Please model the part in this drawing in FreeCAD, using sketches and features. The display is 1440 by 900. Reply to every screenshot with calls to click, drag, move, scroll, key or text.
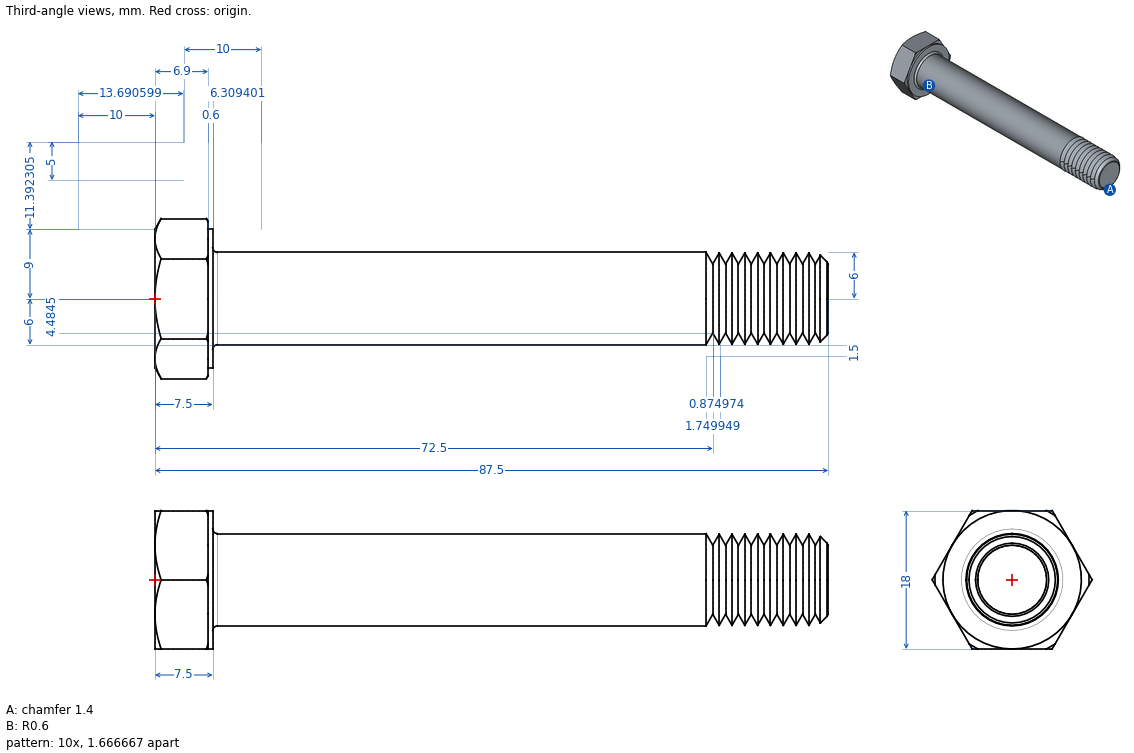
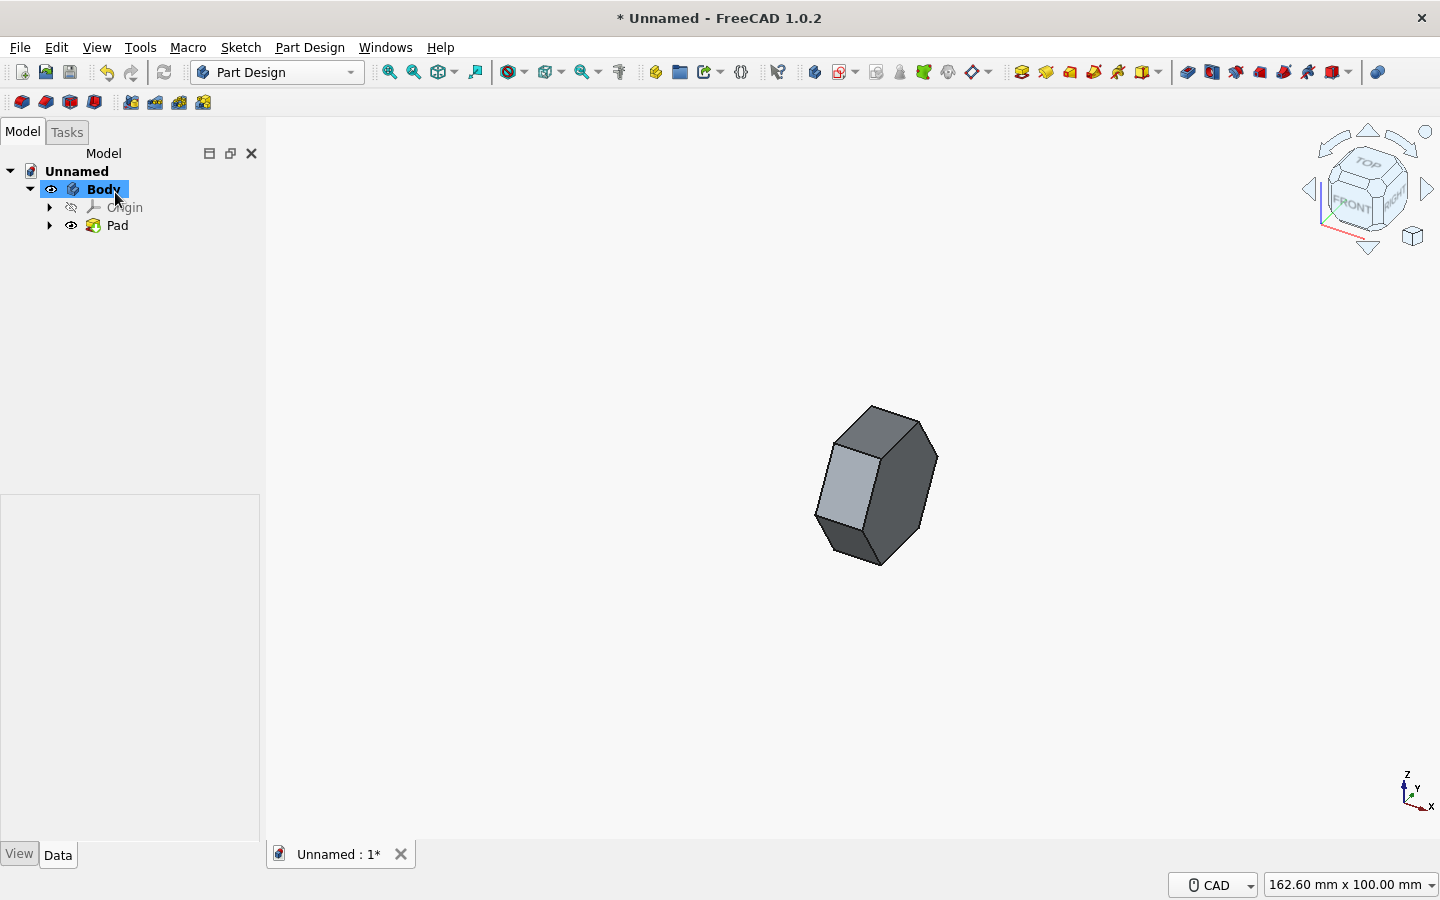
click(390, 72)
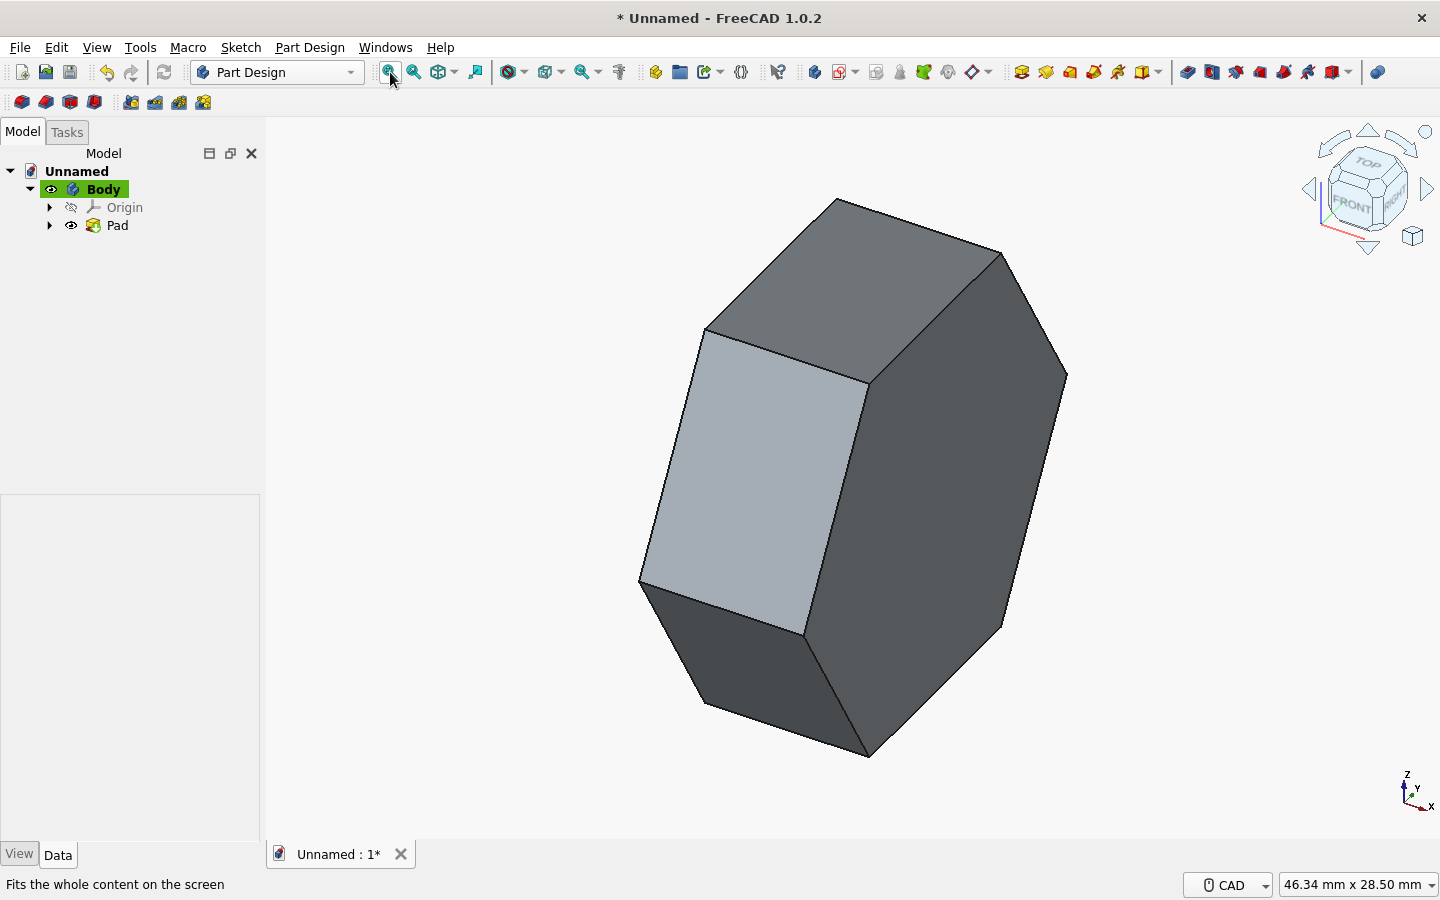
click(840, 72)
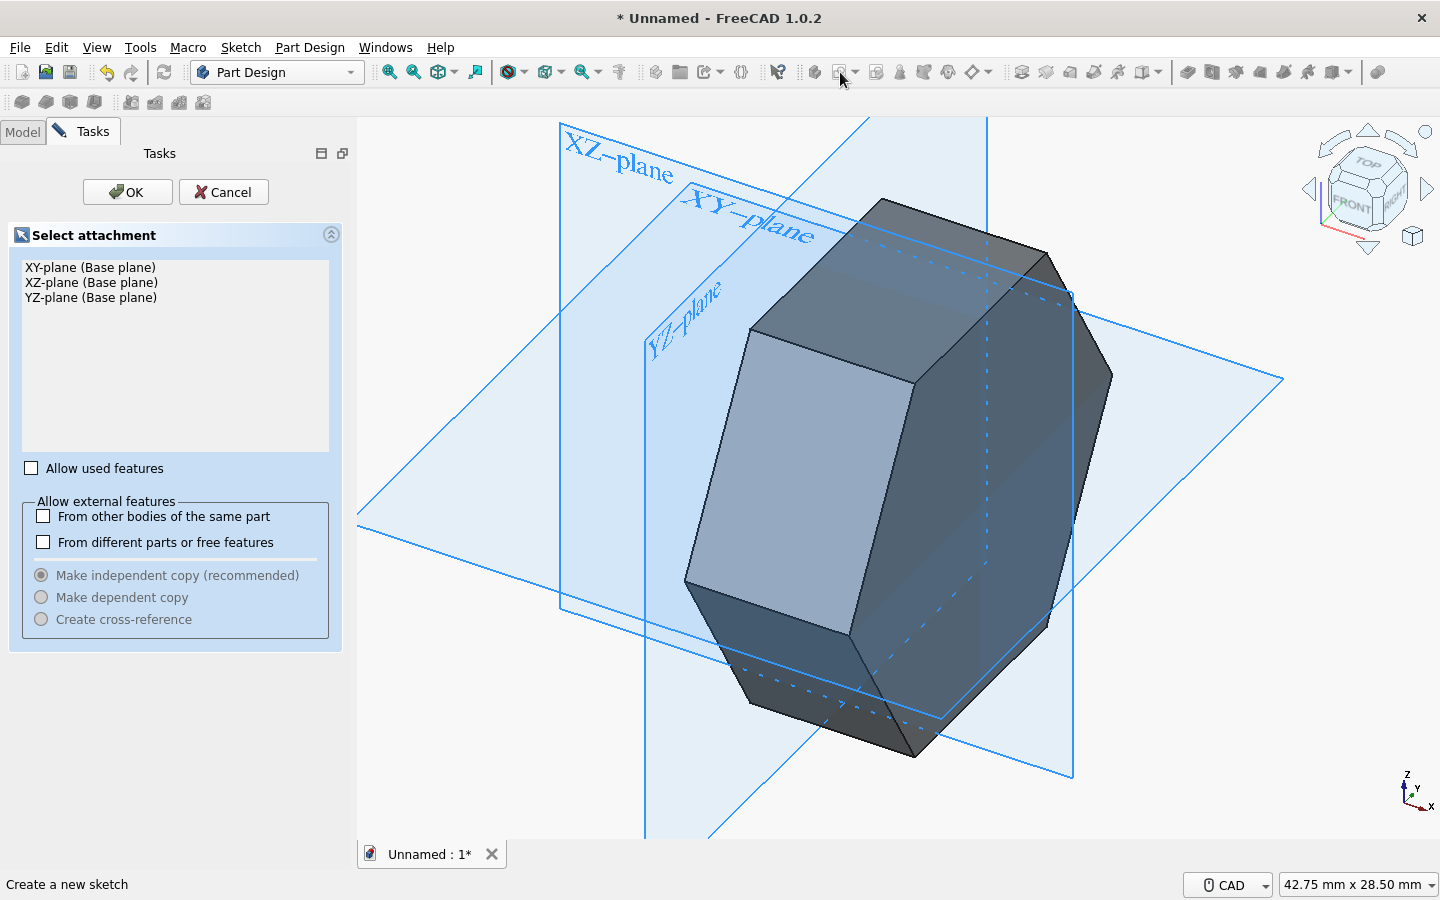
click(82, 268)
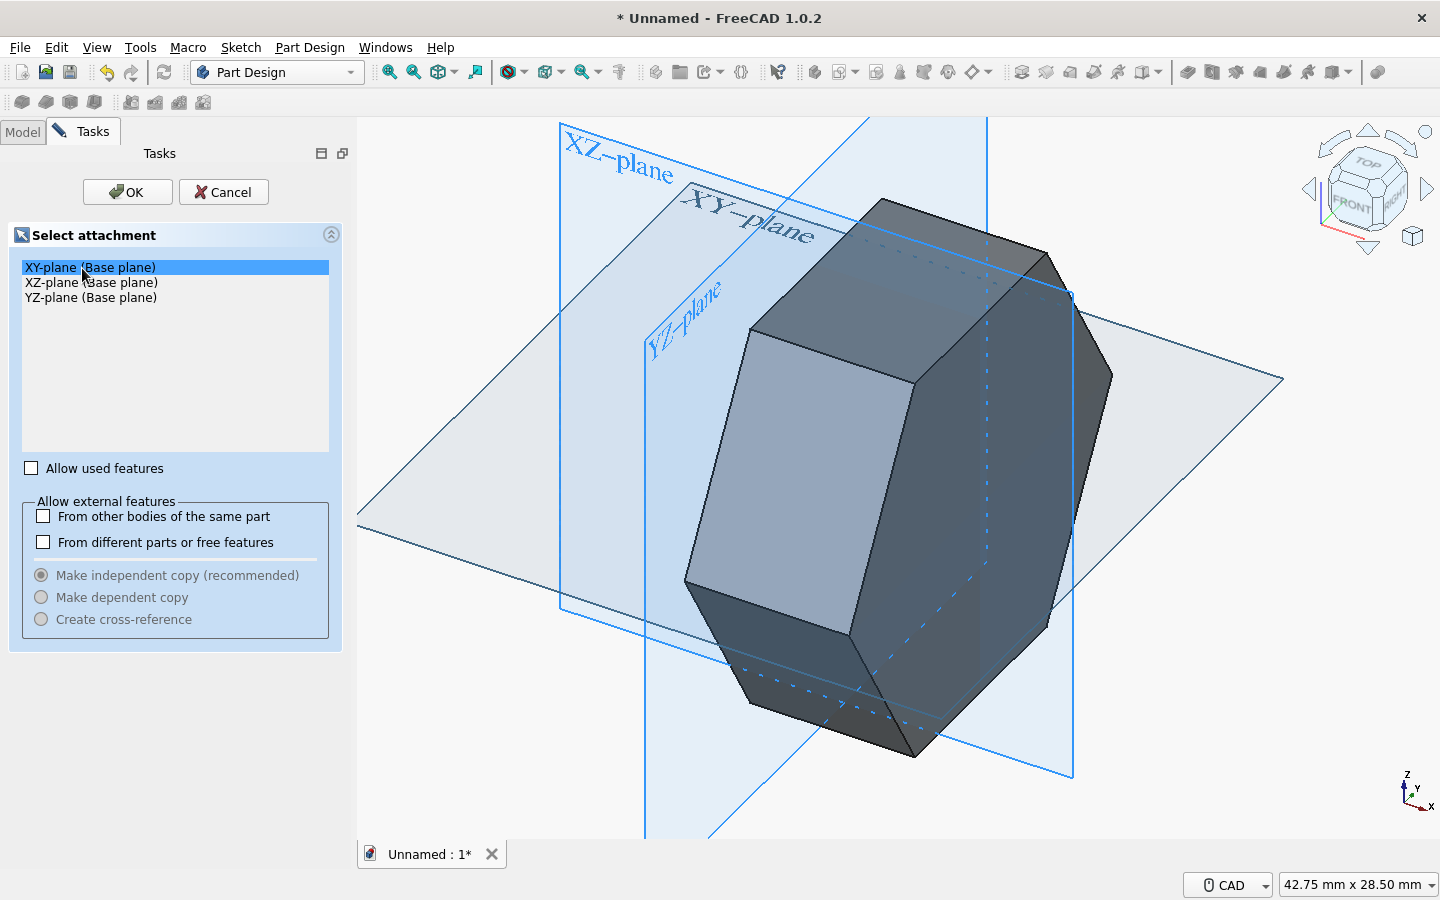
click(128, 192)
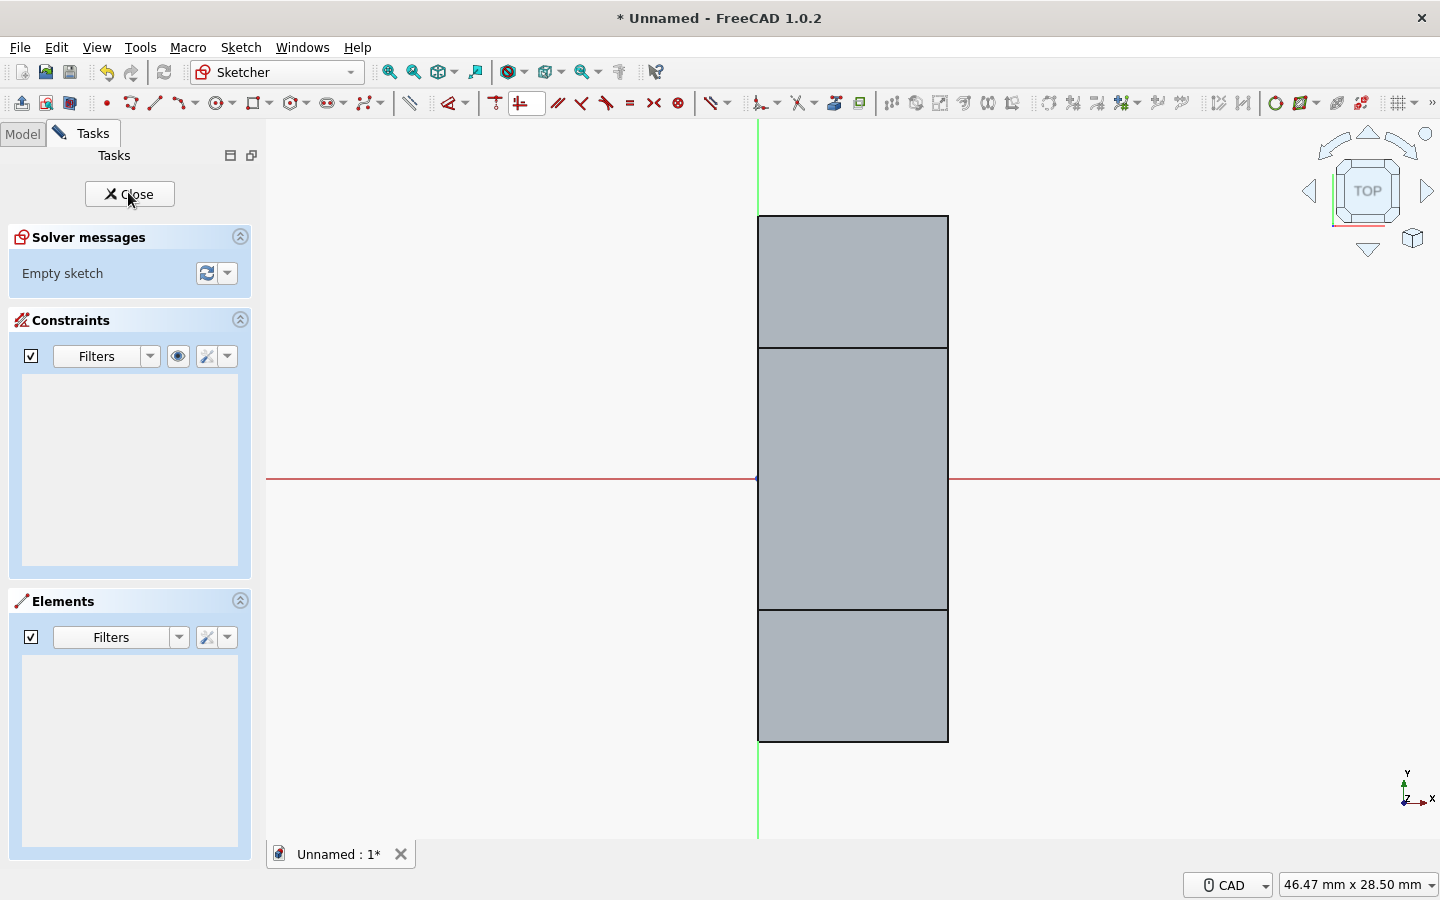
click(70, 104)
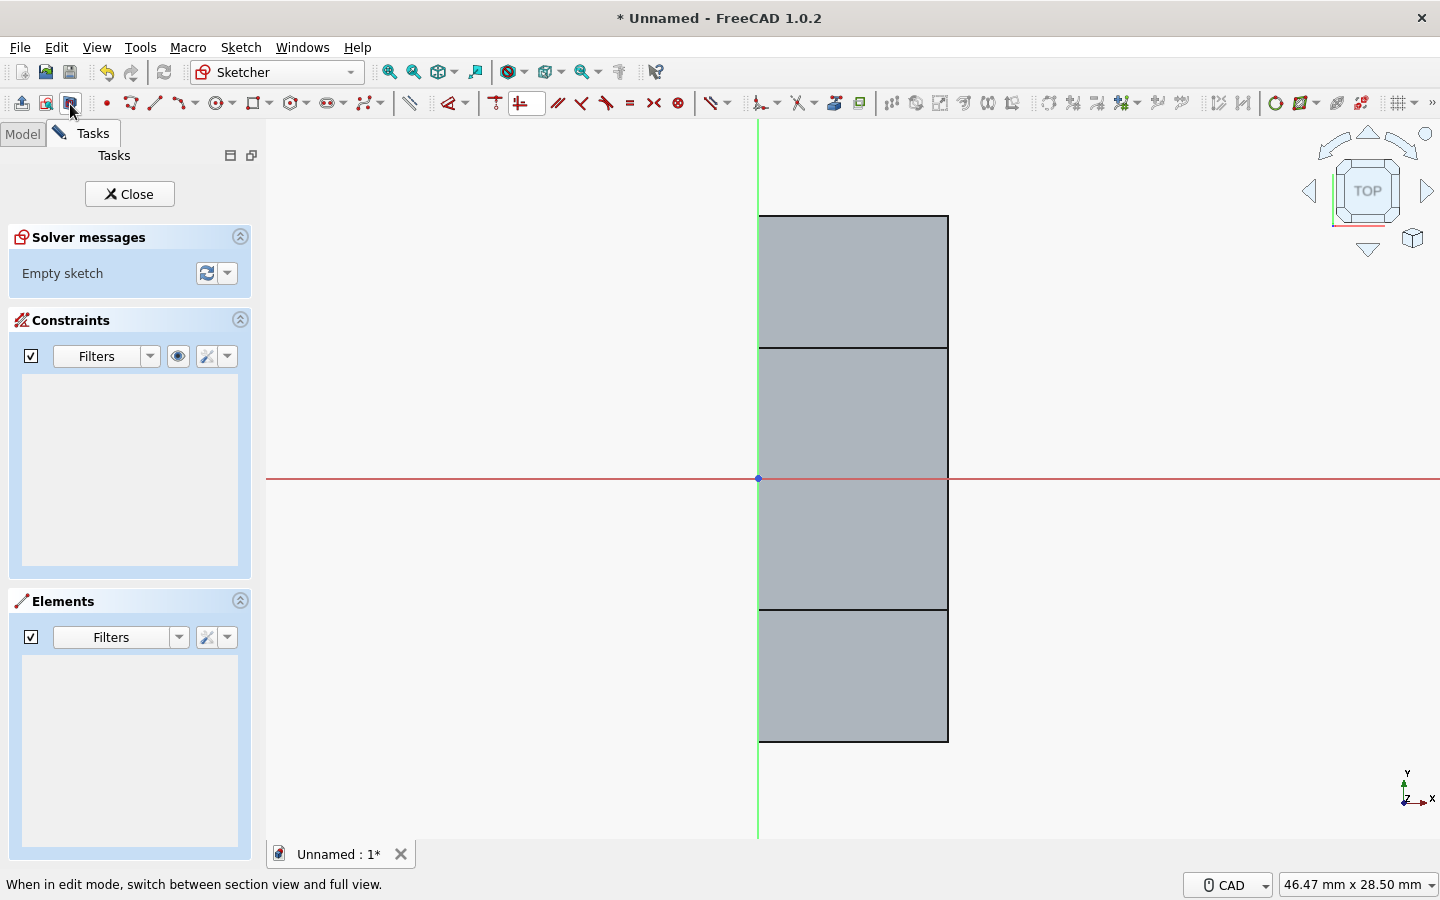
scroll(319, 512, down, 6)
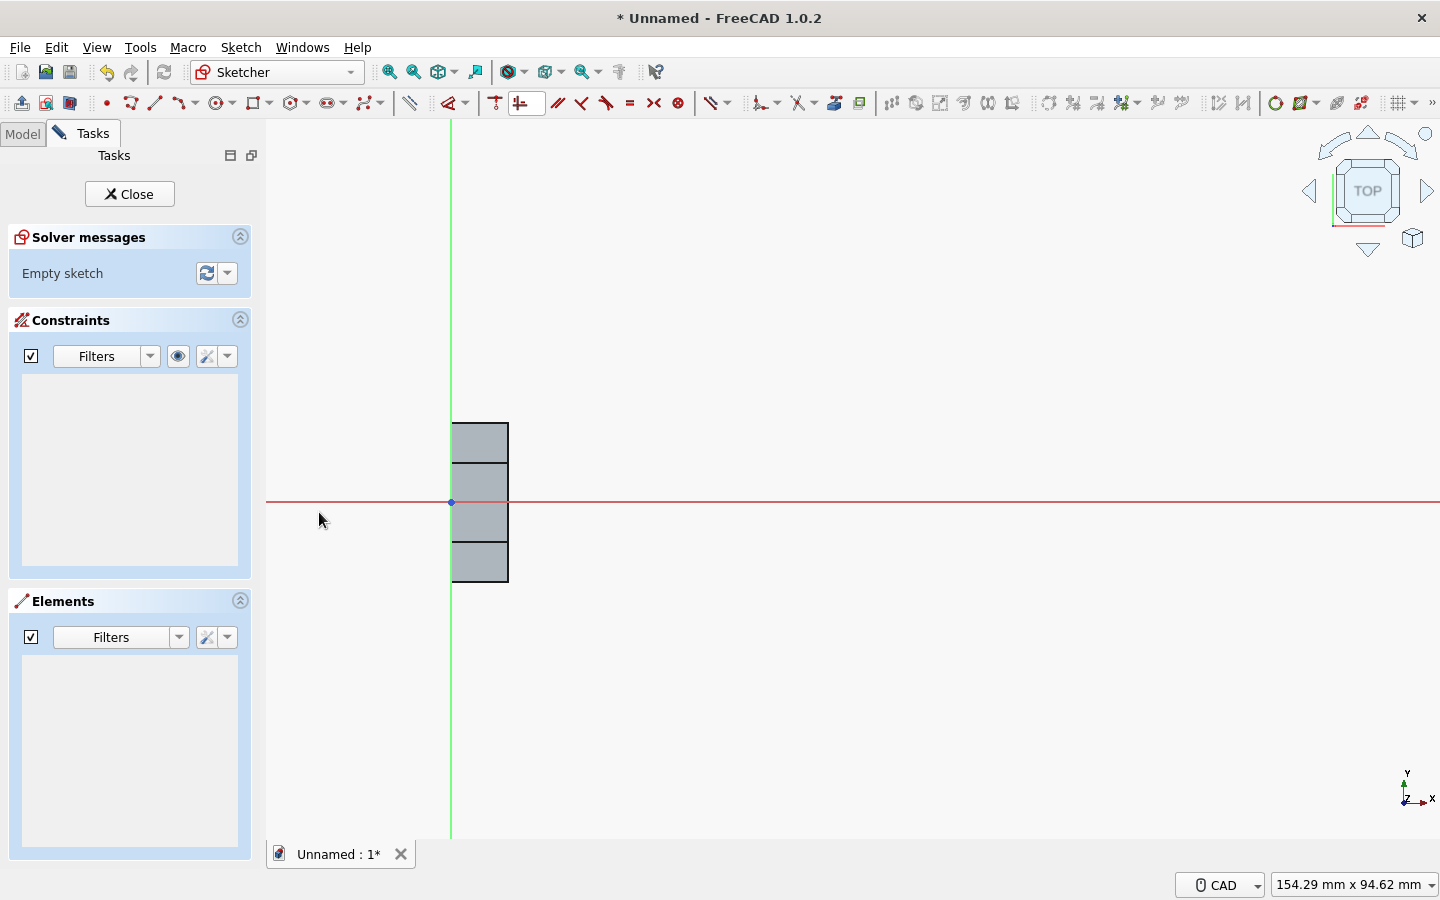
click(254, 104)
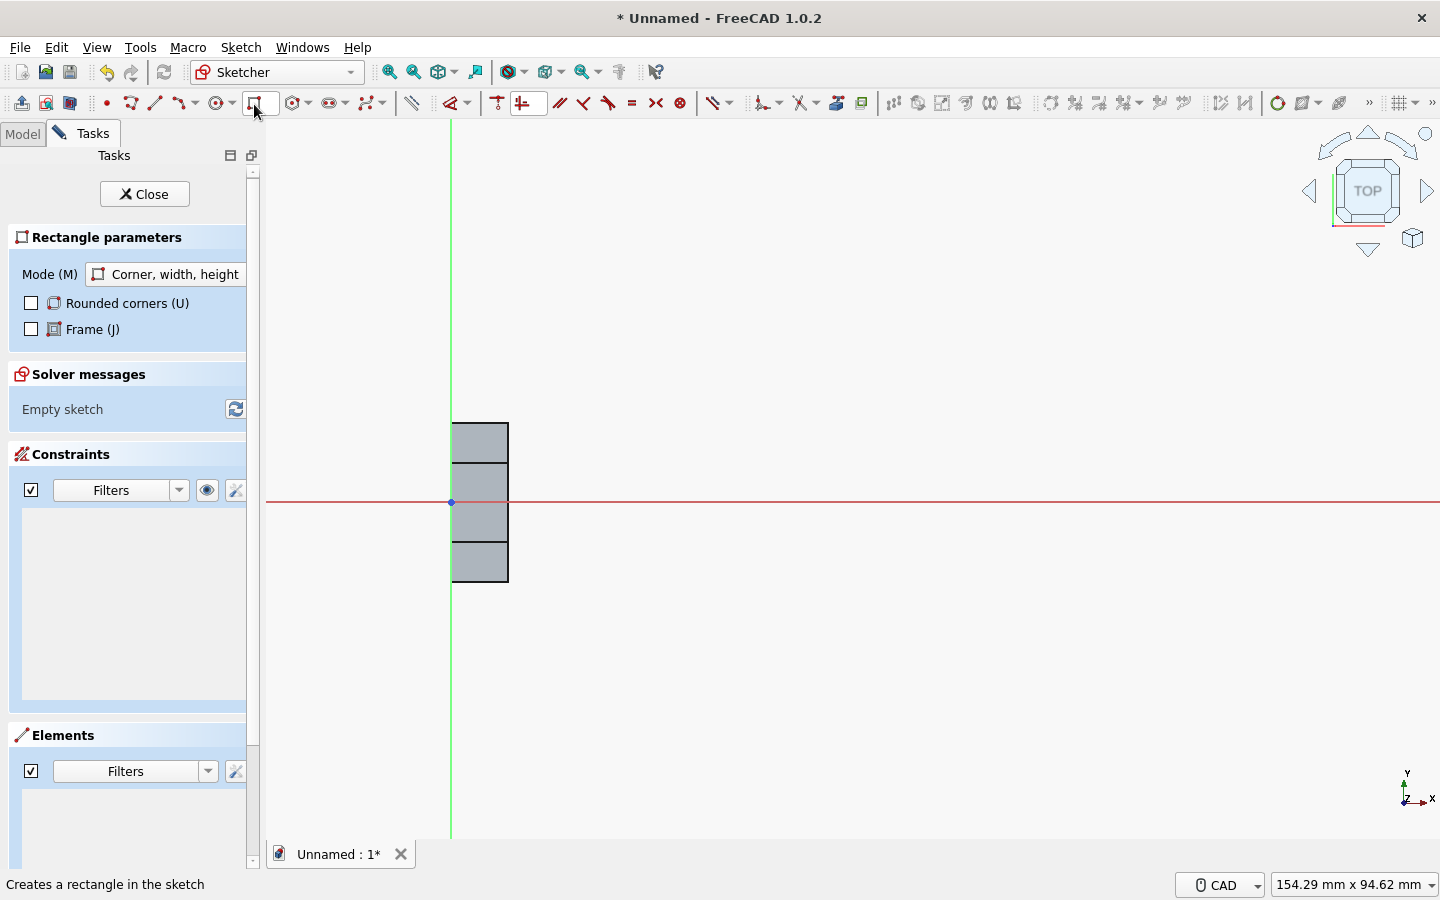
click(451, 502)
click(1117, 457)
key(Escape)